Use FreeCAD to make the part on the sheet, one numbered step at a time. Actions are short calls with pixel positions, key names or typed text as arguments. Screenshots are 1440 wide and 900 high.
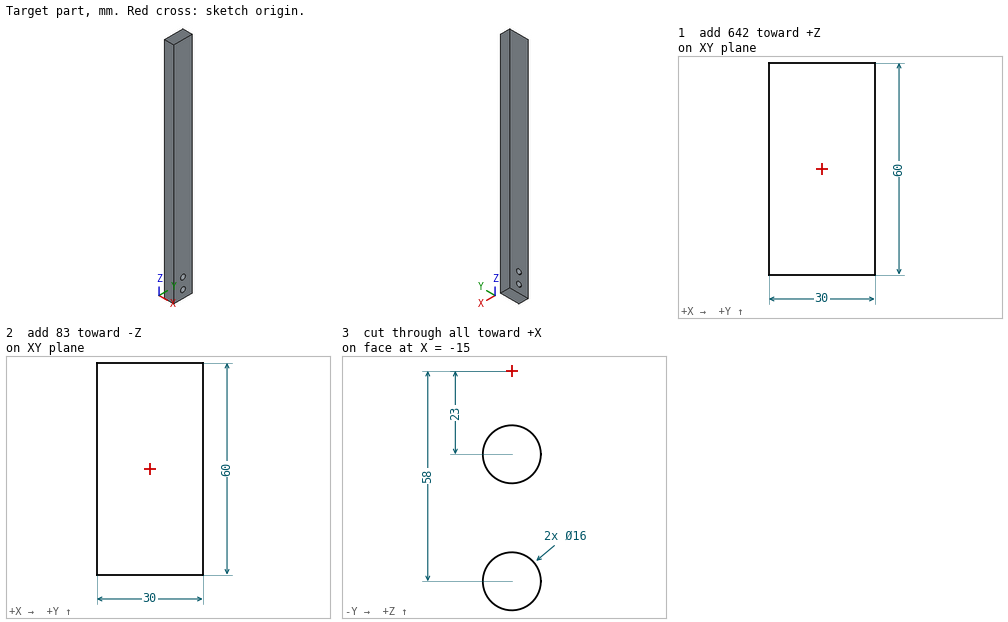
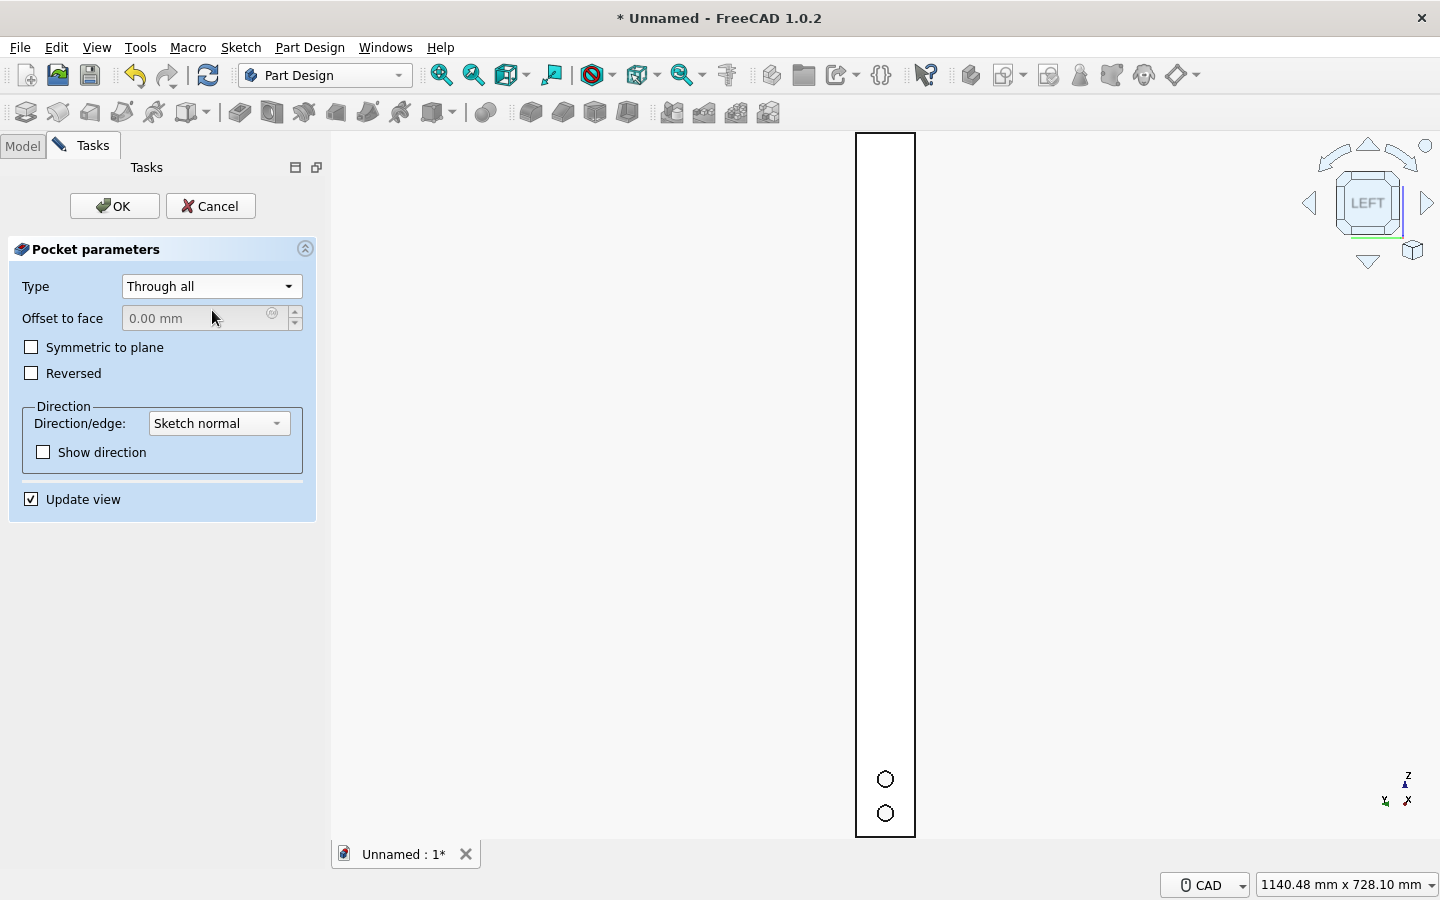
click(115, 206)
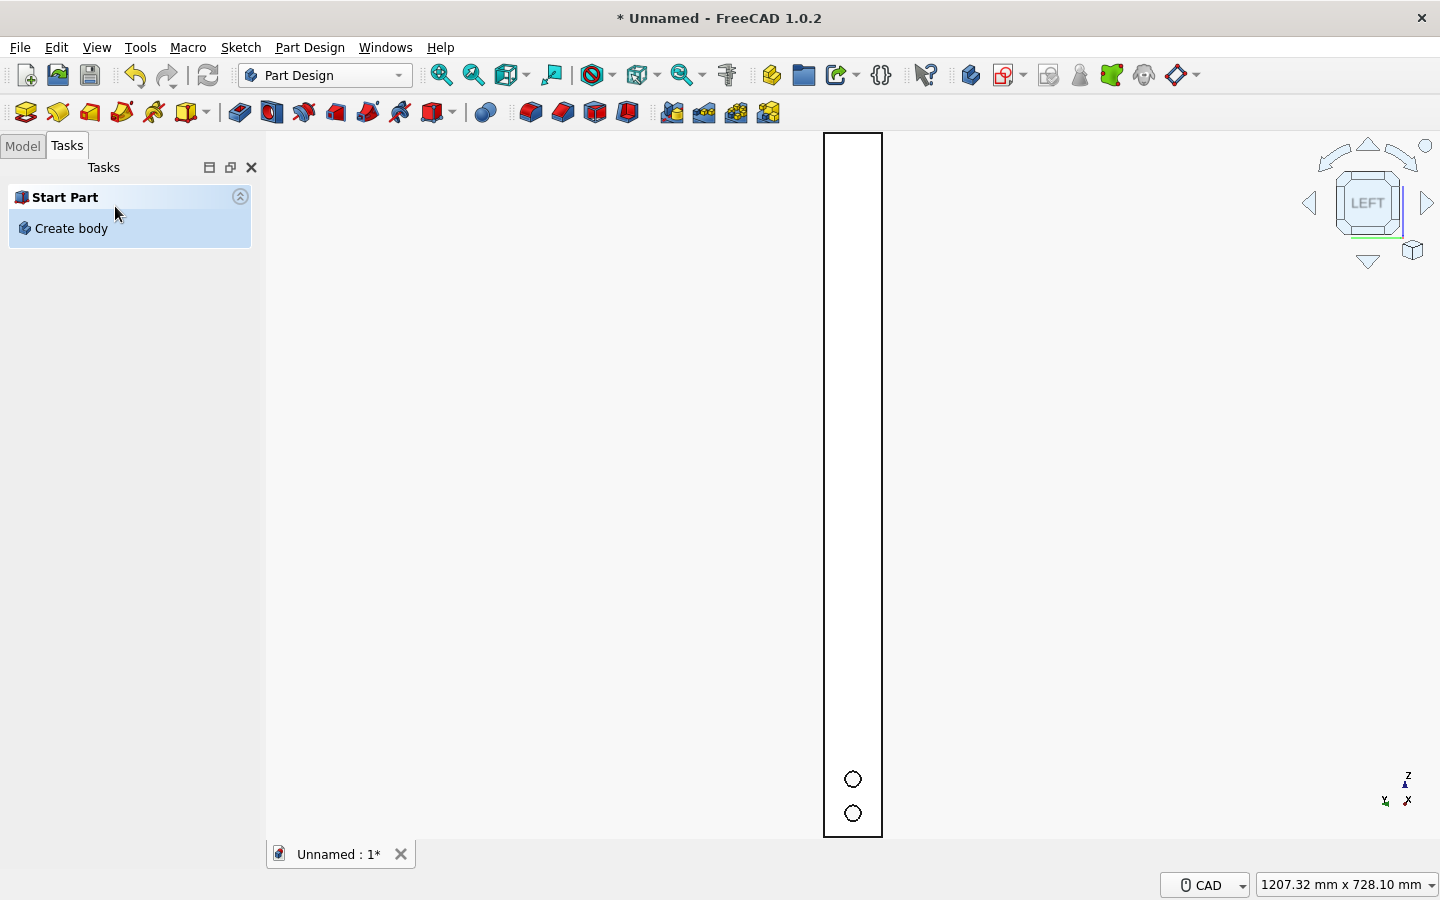
key(0)